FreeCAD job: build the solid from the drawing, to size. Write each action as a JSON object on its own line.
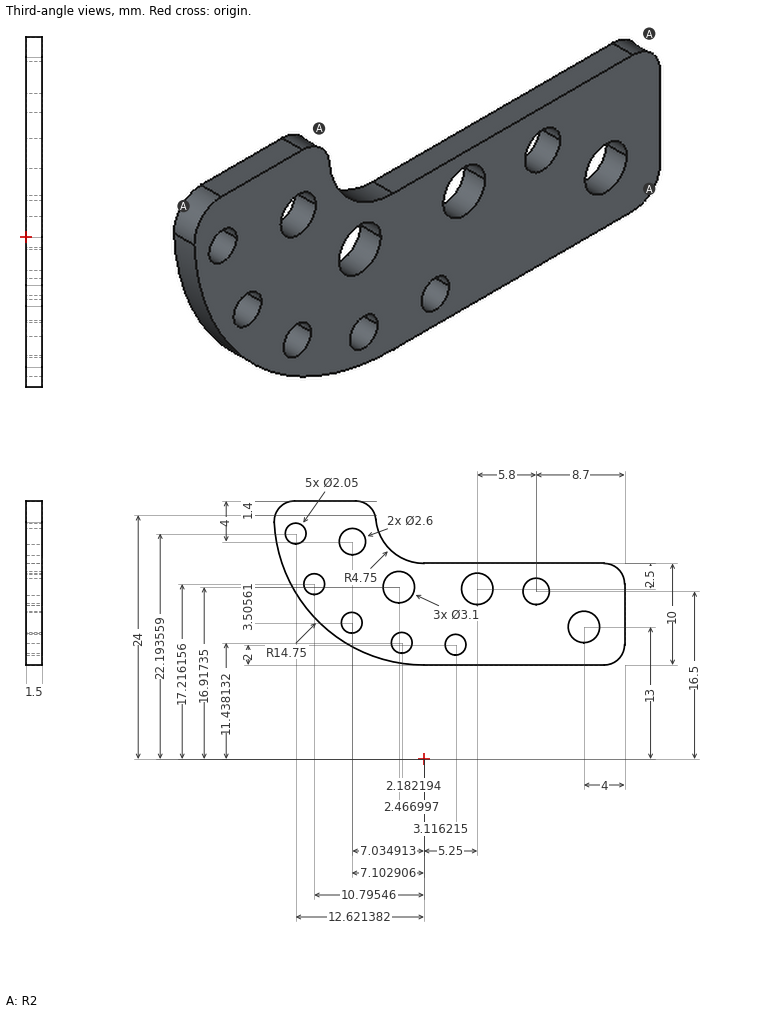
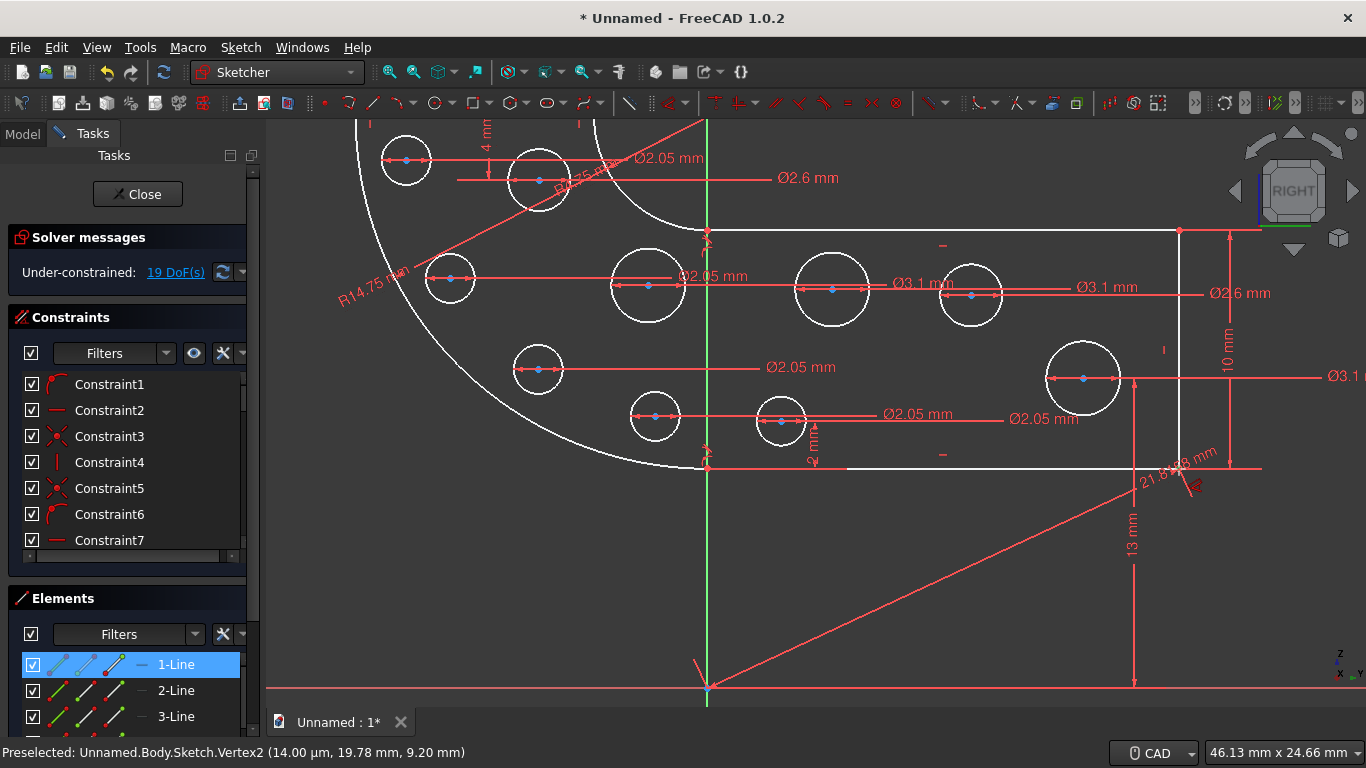
{"action": "left_click", "coordinate": [1083, 378]}
{"action": "left_click", "coordinate": [1131, 503]}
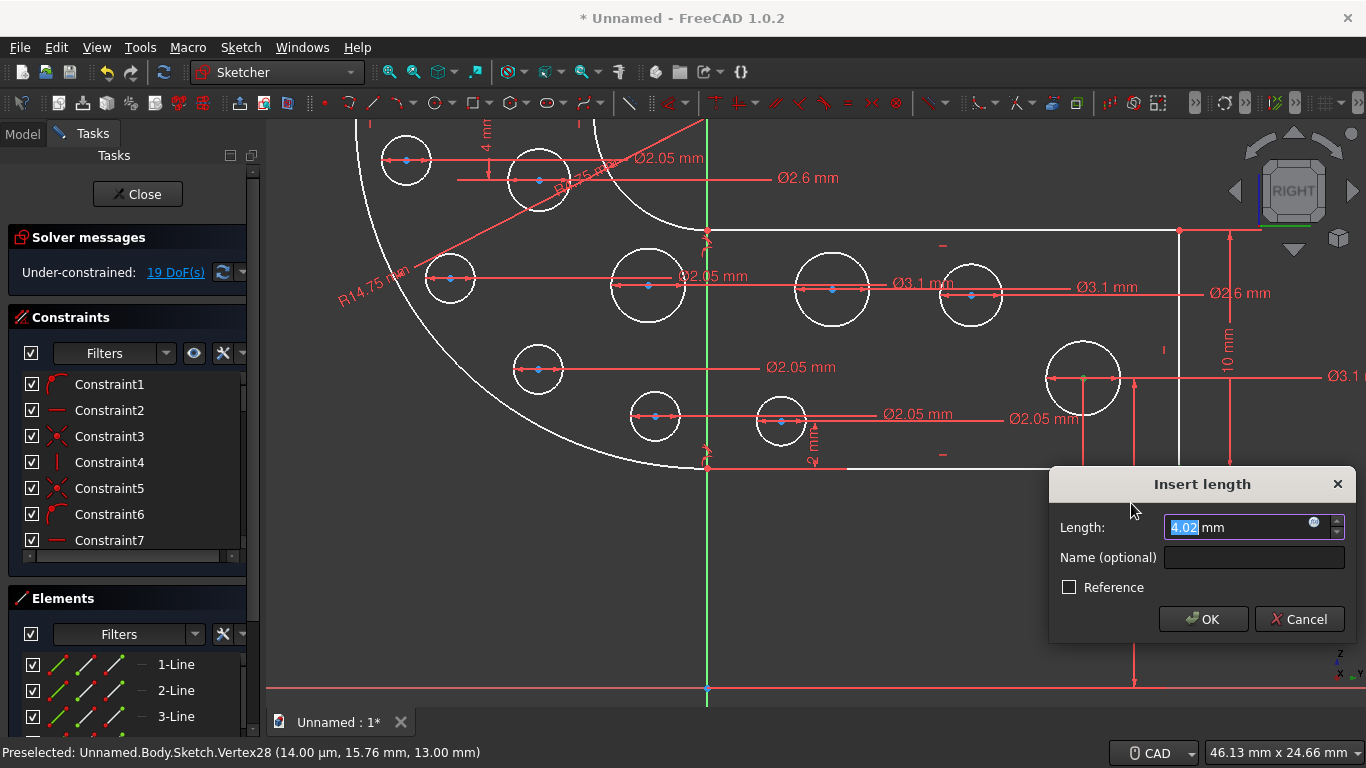
{"action": "type", "text": "4"}
{"action": "key", "text": "Return"}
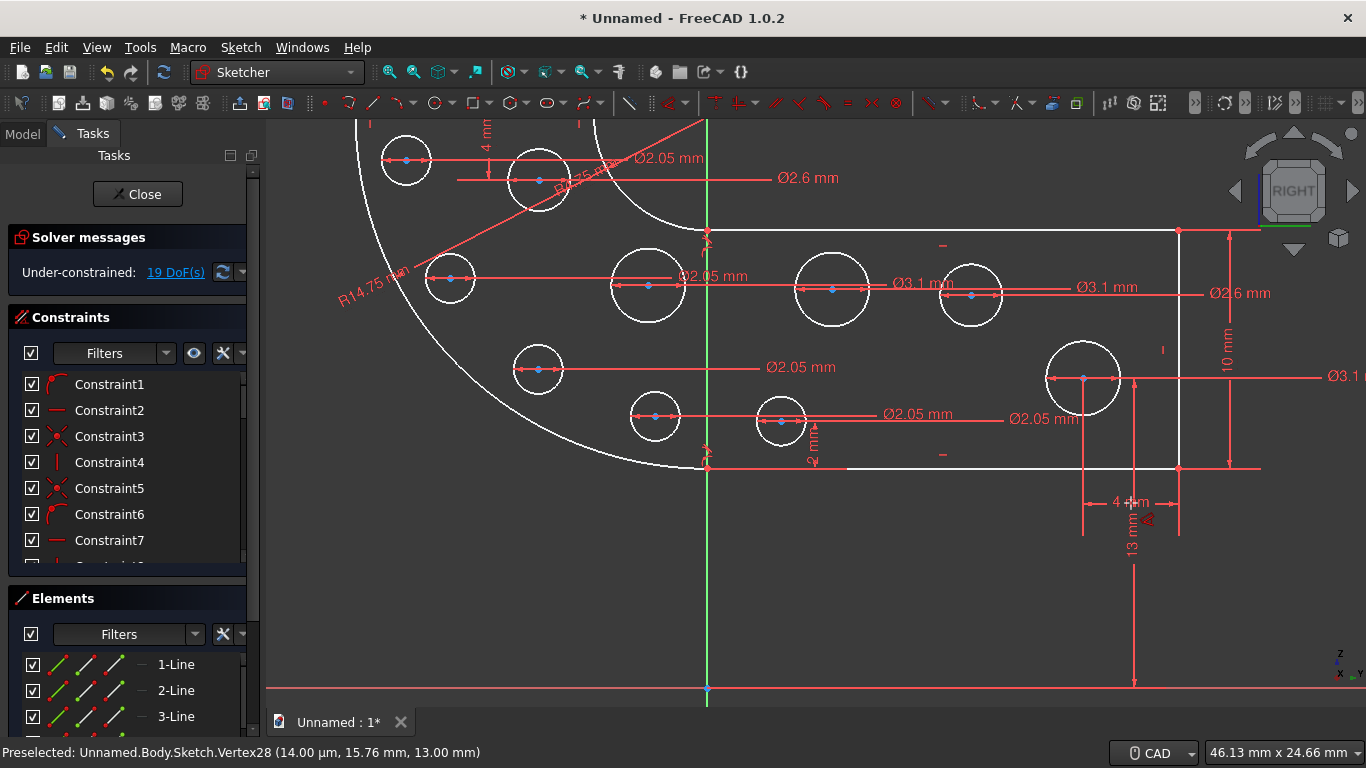
{"action": "scroll", "coordinate": [708, 469], "scroll_direction": "down", "scroll_amount": 2}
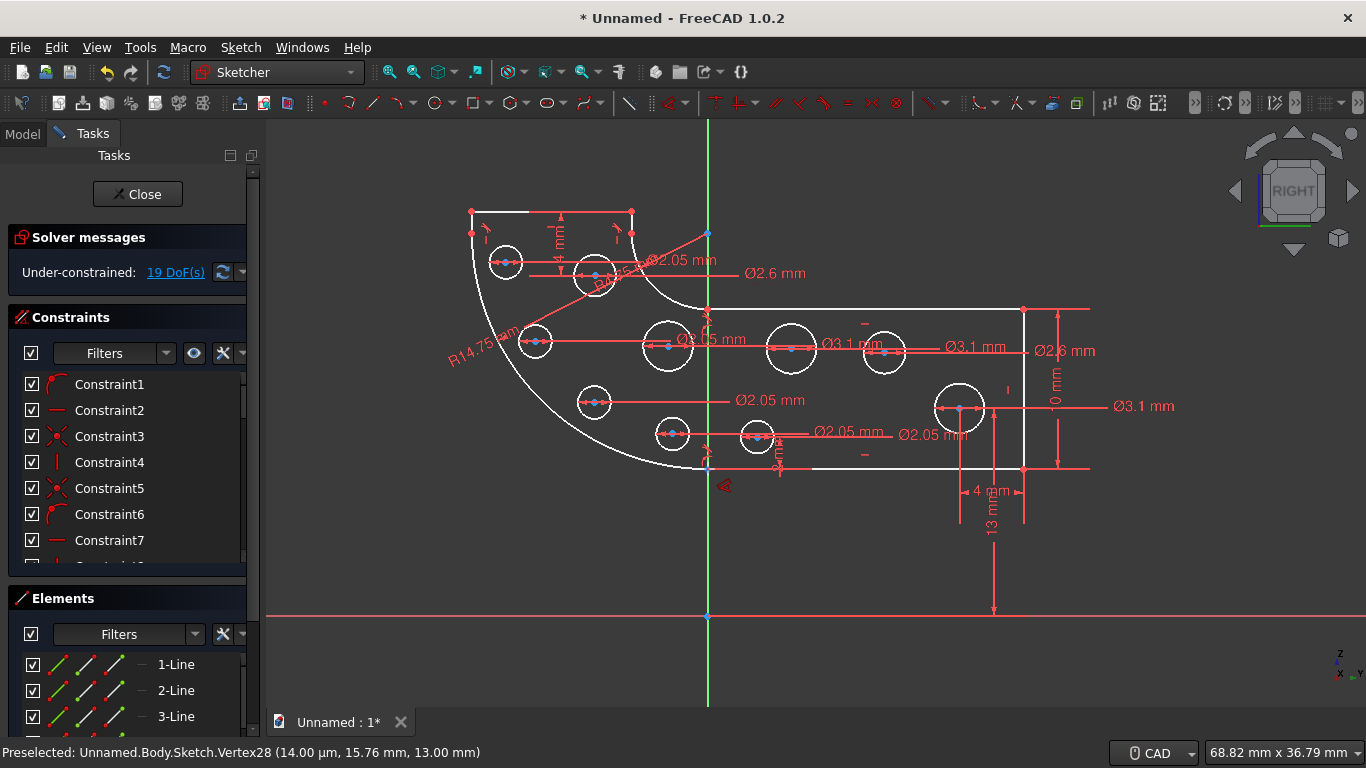
{"action": "scroll", "coordinate": [632, 227], "scroll_direction": "up", "scroll_amount": 4}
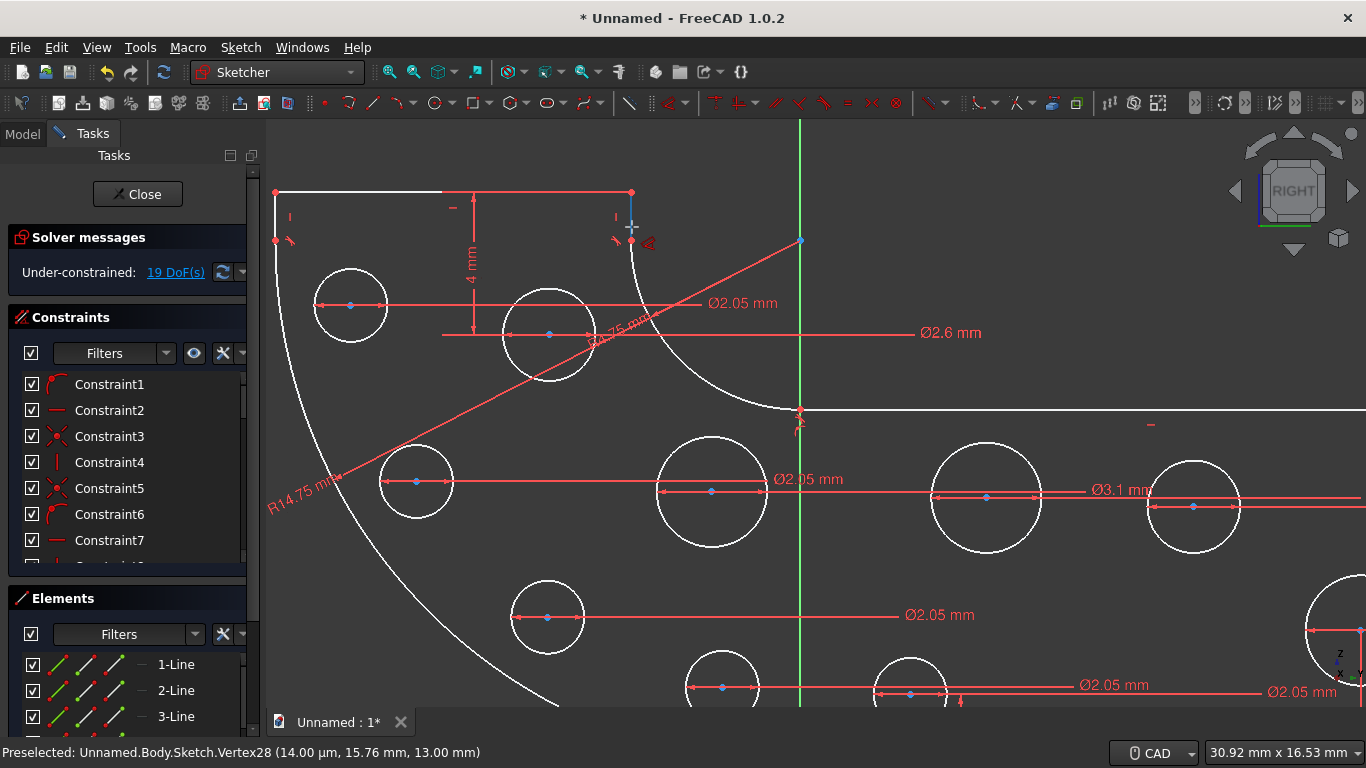
{"action": "left_click", "coordinate": [631, 226]}
{"action": "left_click", "coordinate": [597, 217]}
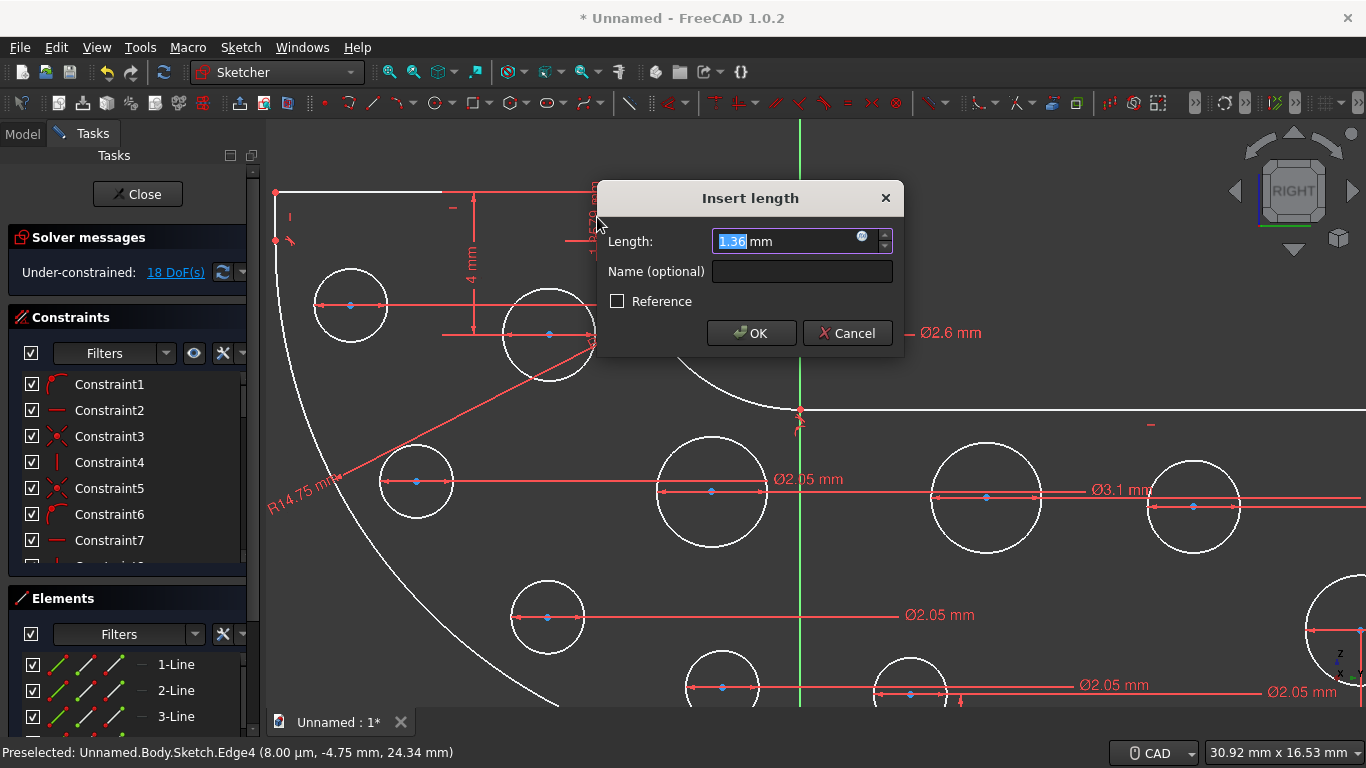
{"action": "type", "text": "1.4"}
{"action": "key", "text": "Return"}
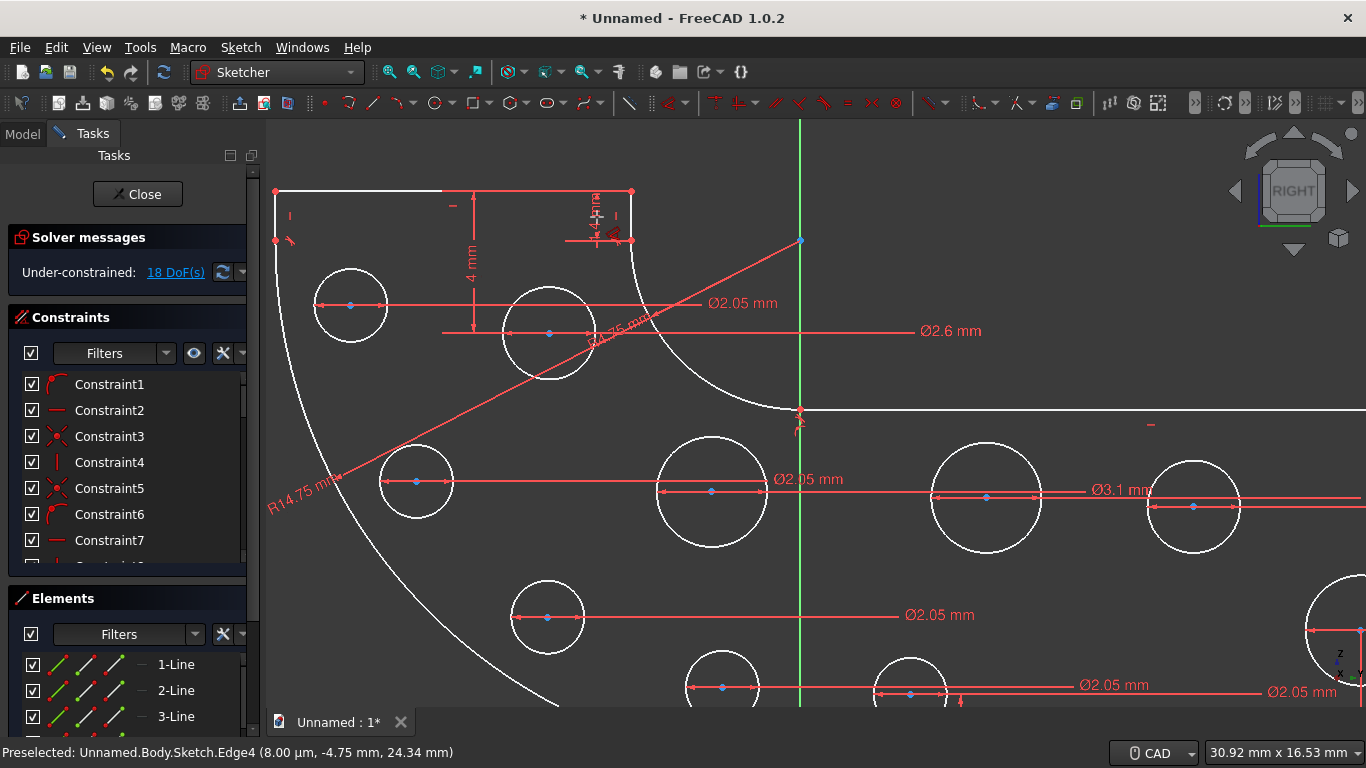
{"action": "left_click", "coordinate": [631, 241]}
{"action": "left_click", "coordinate": [597, 460]}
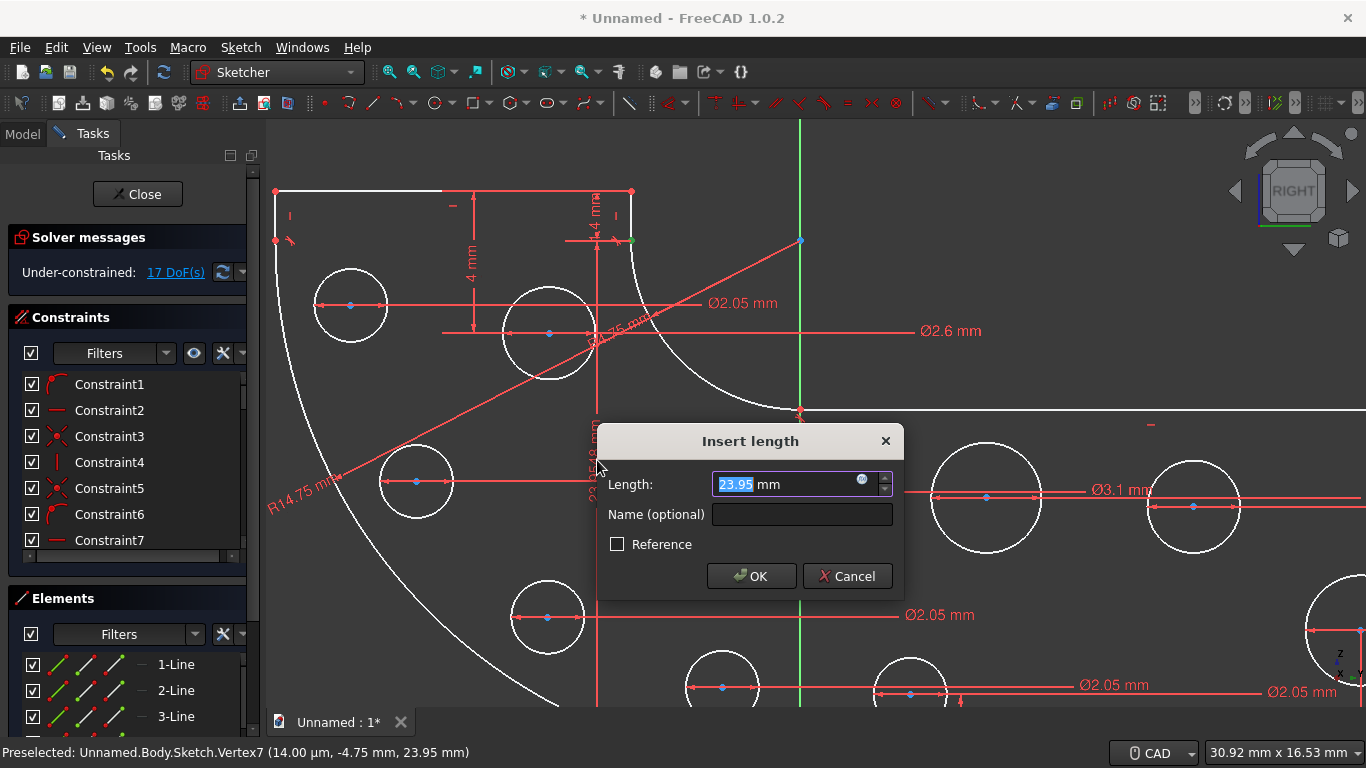
{"action": "type", "text": "24"}
{"action": "key", "text": "Return"}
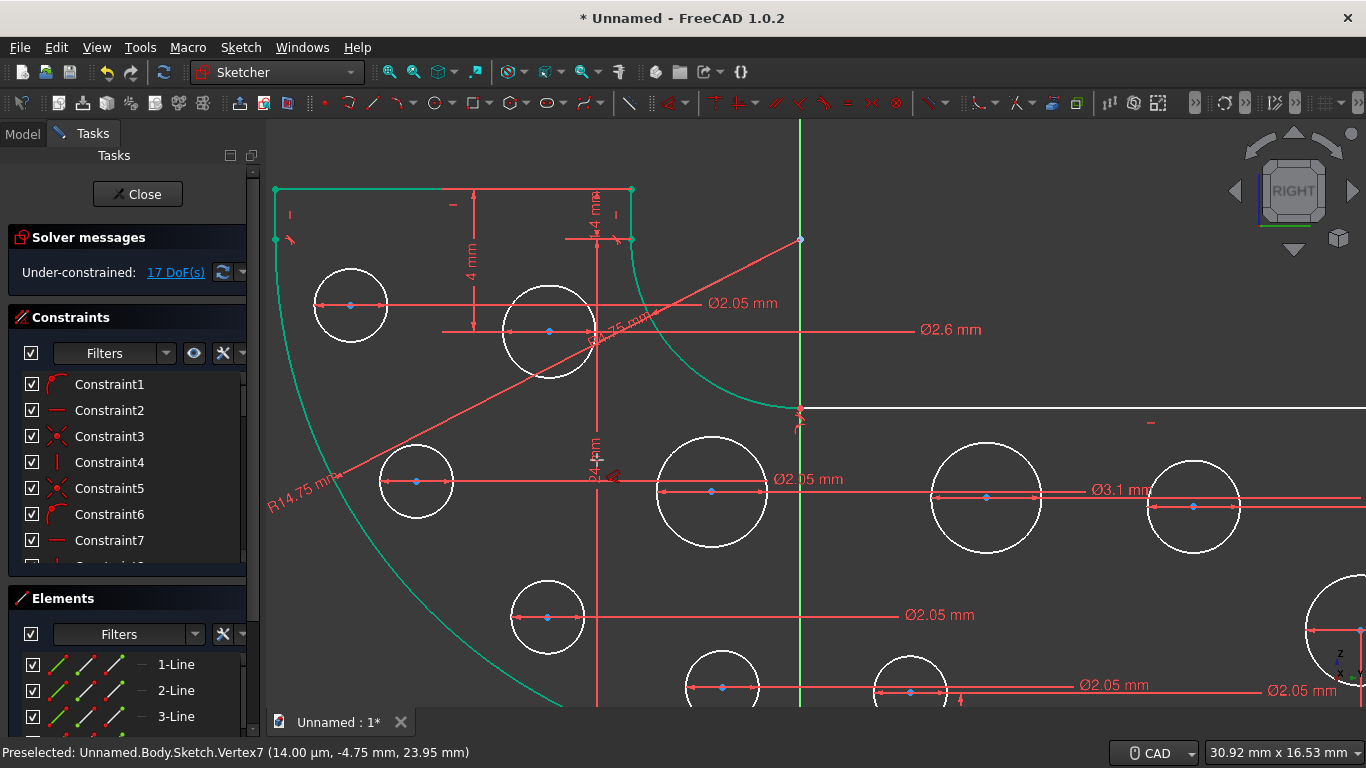
{"action": "left_click", "coordinate": [986, 498]}
{"action": "left_click", "coordinate": [893, 464]}